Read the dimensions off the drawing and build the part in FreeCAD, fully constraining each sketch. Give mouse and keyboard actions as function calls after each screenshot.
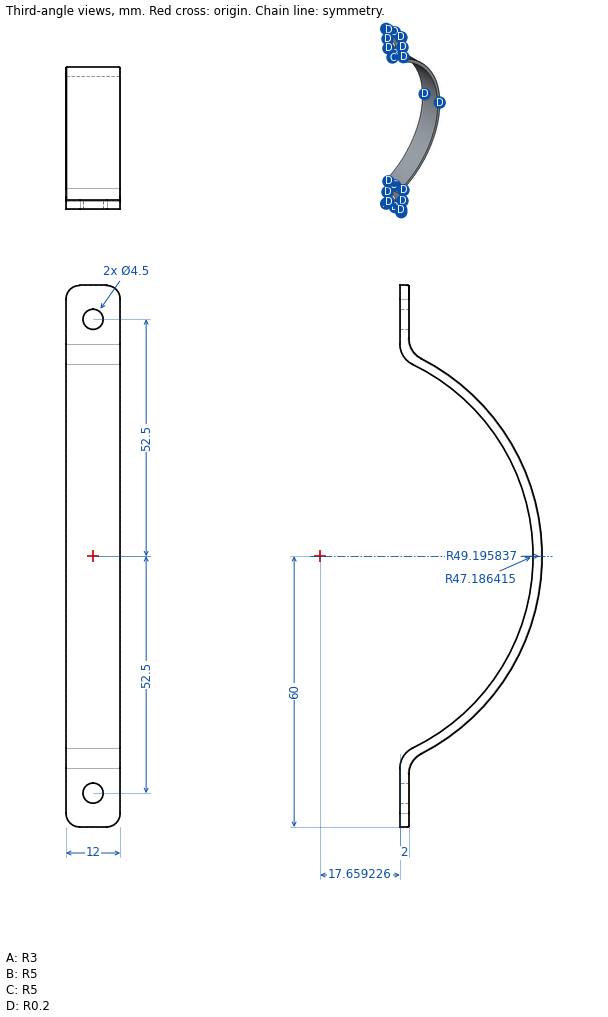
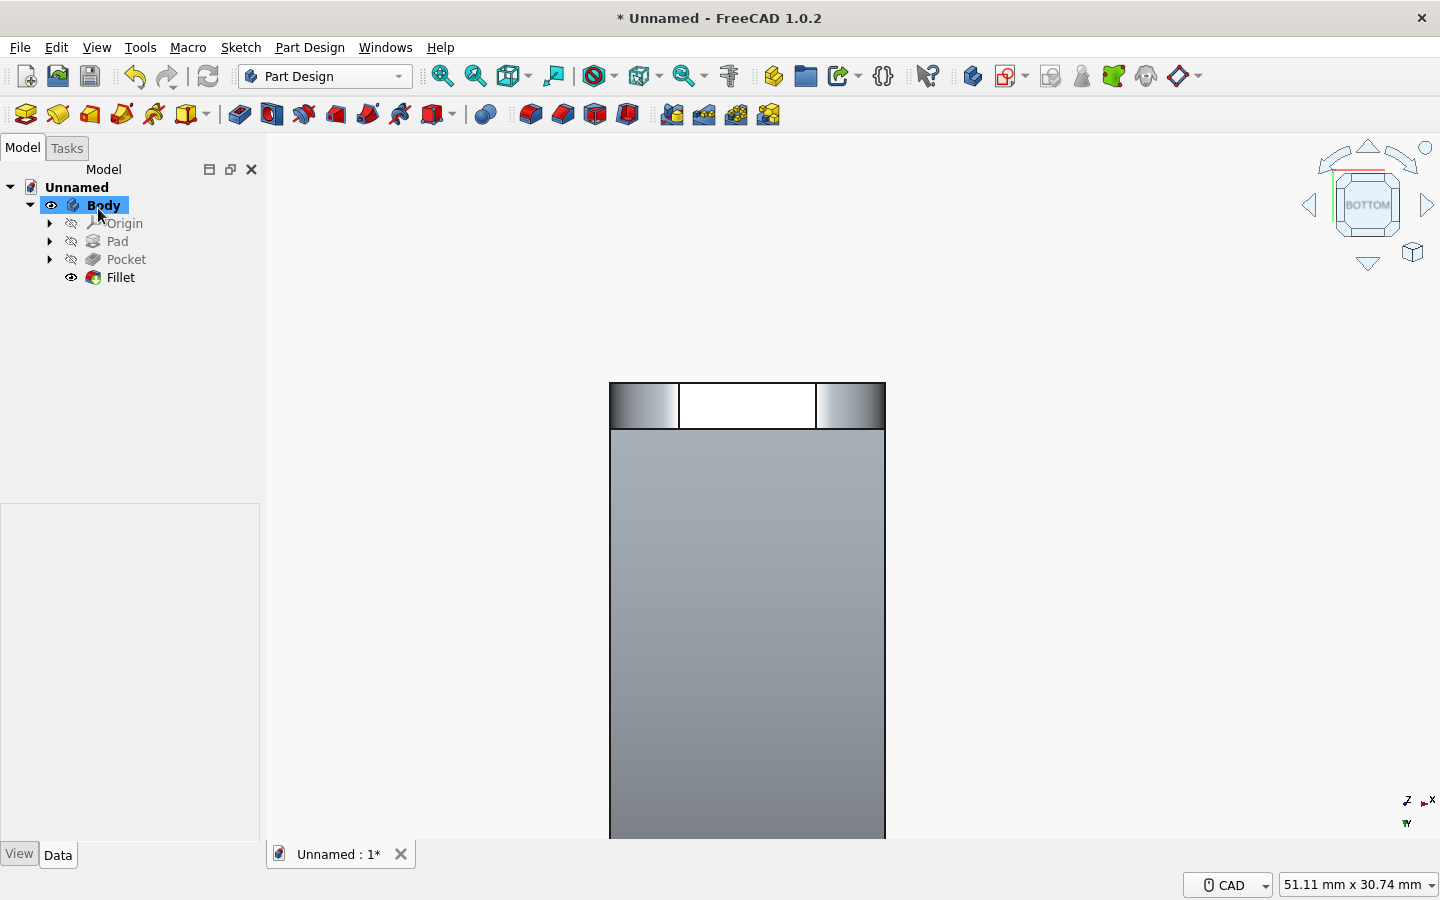
click(444, 76)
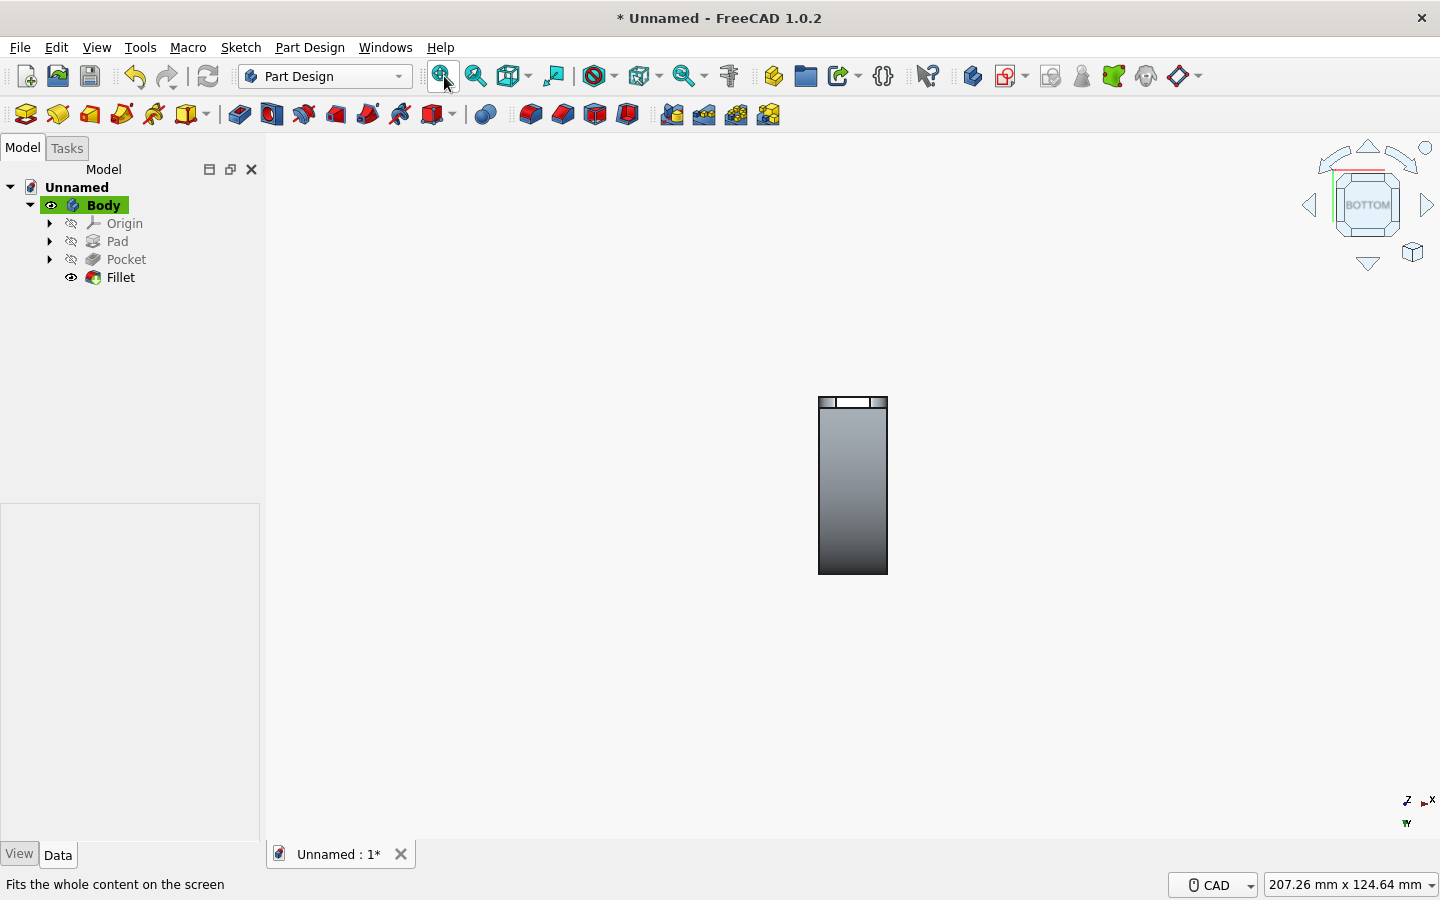
key(0)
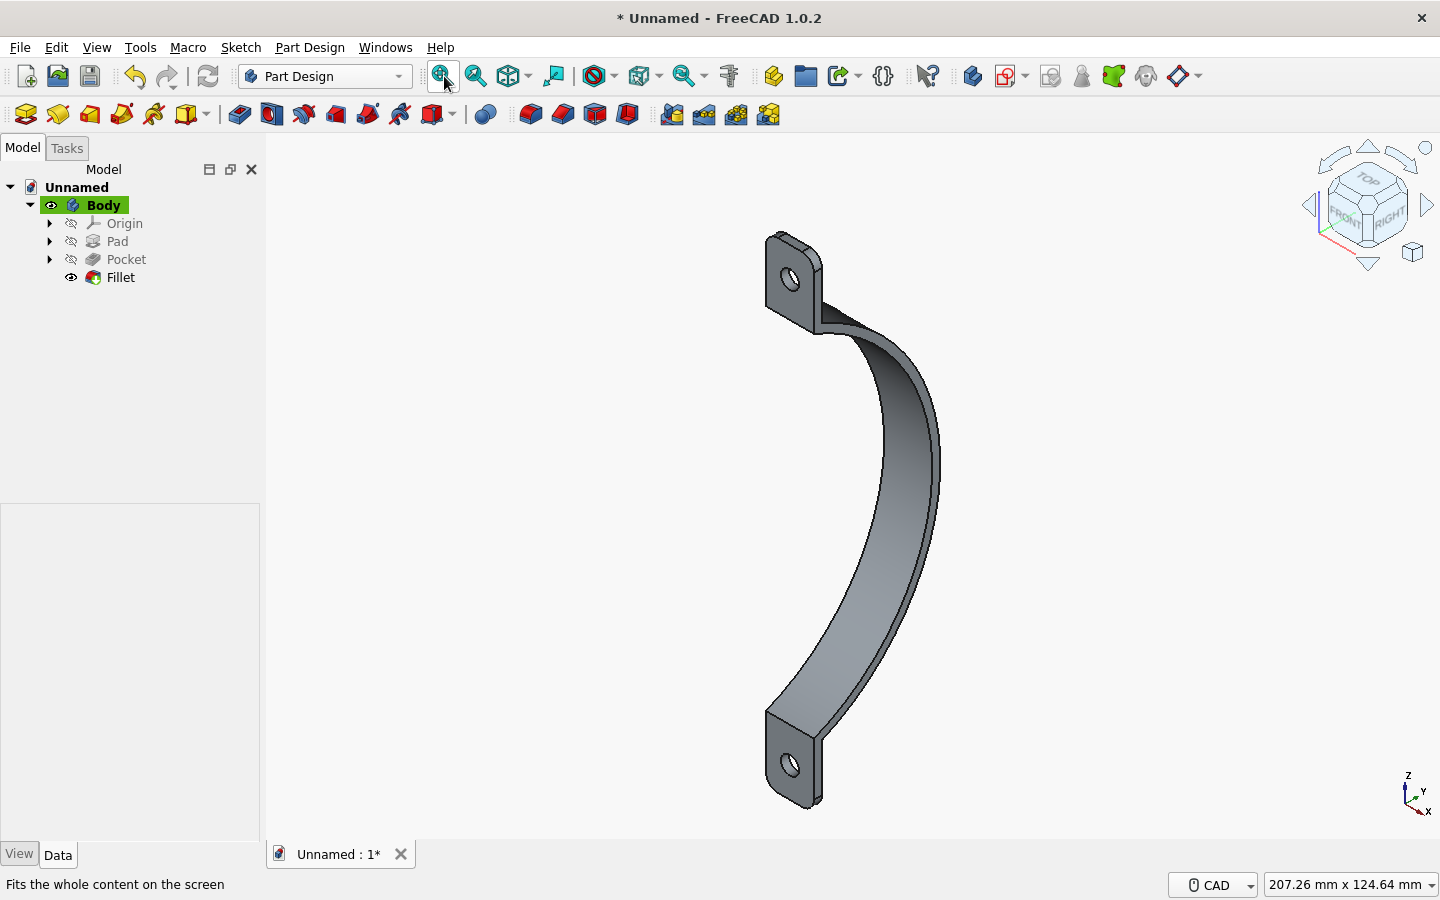
key(2)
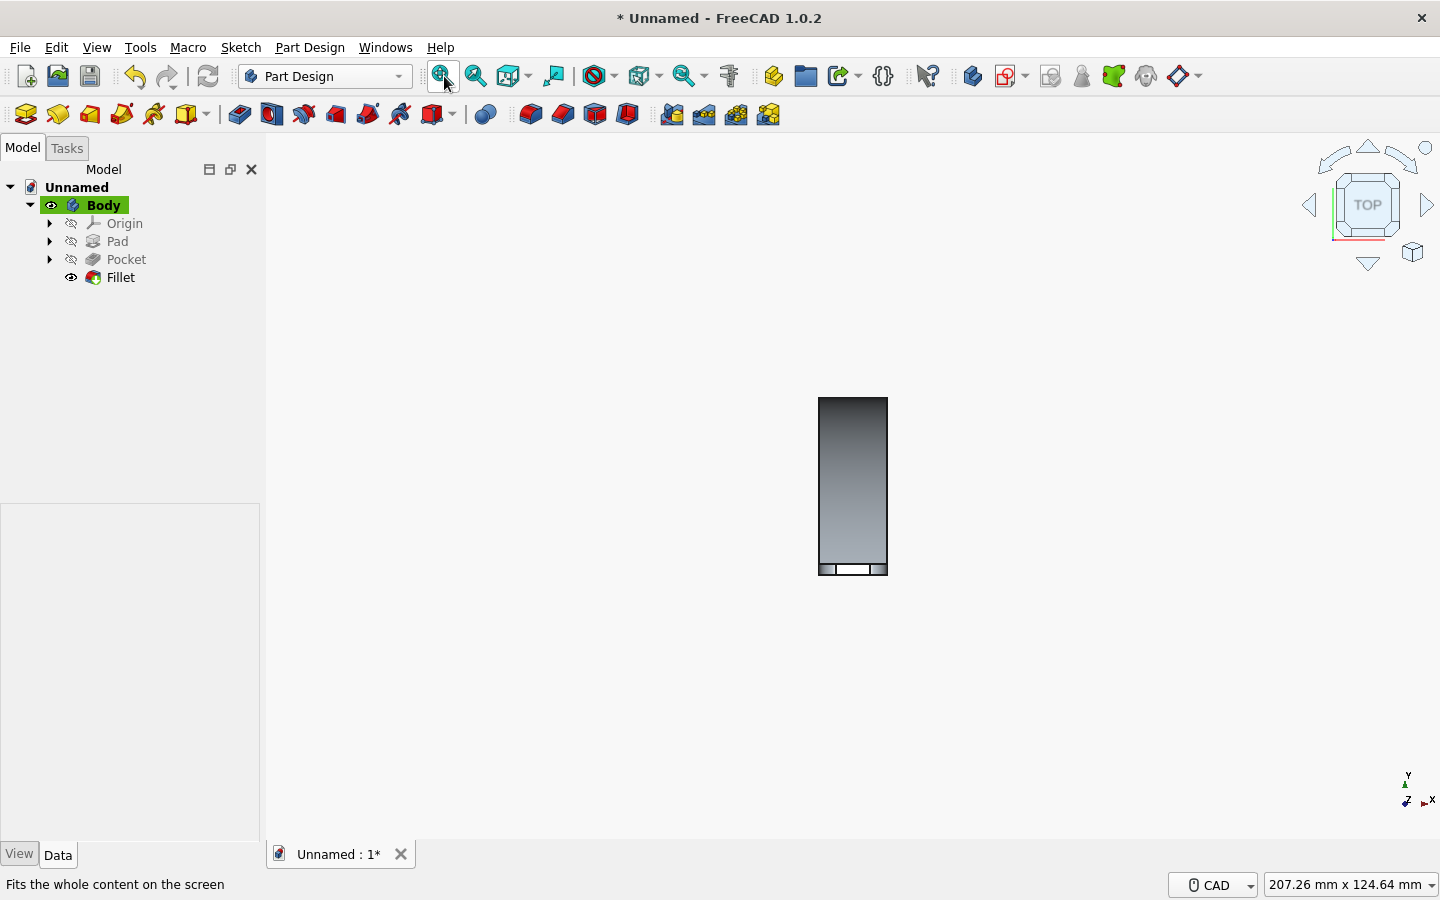
key(v)
key(f)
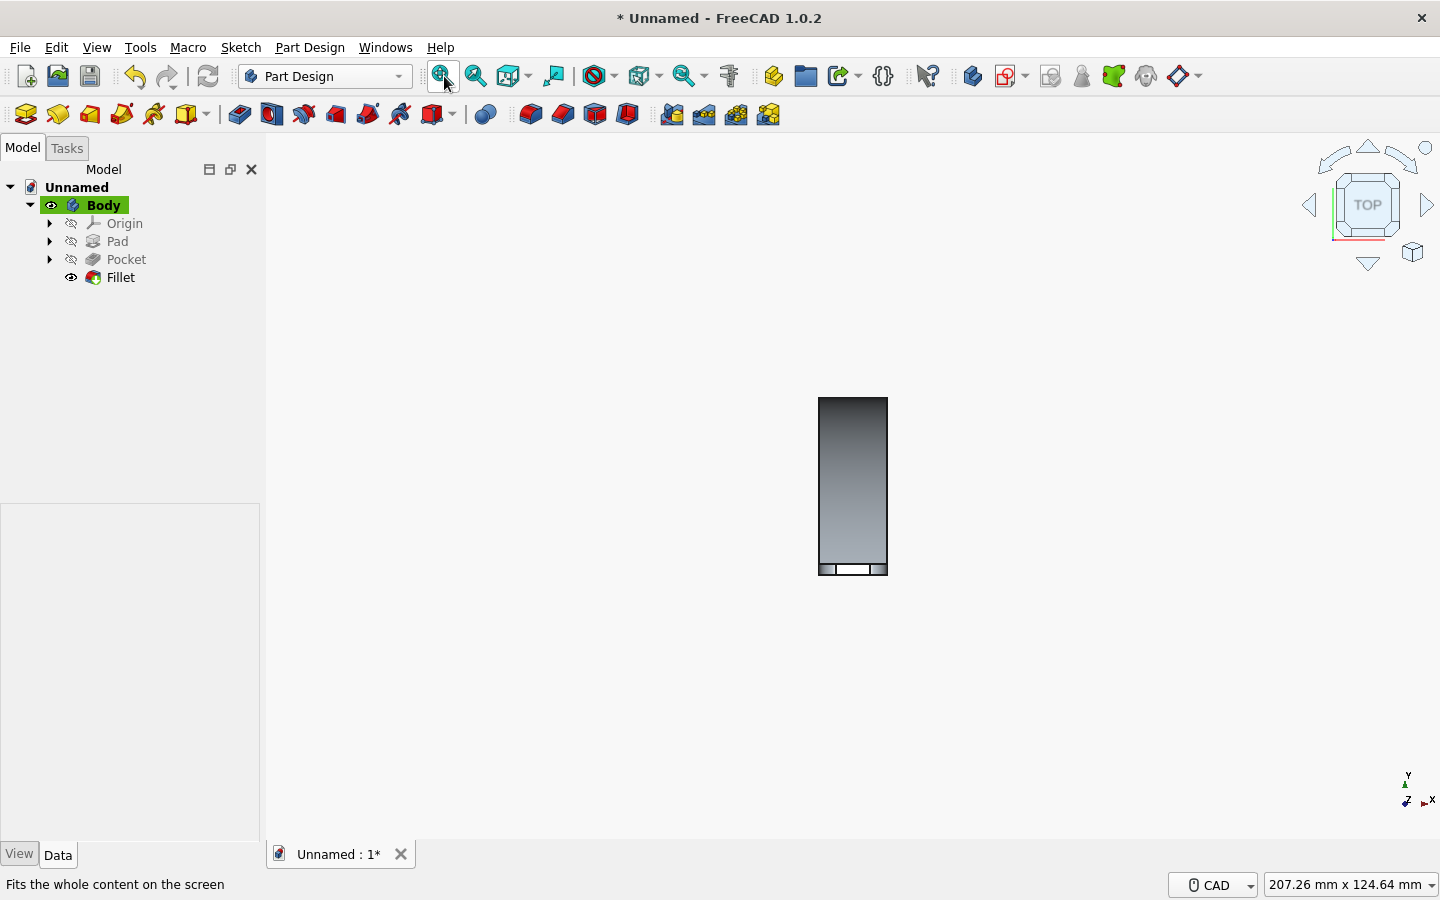
key(1)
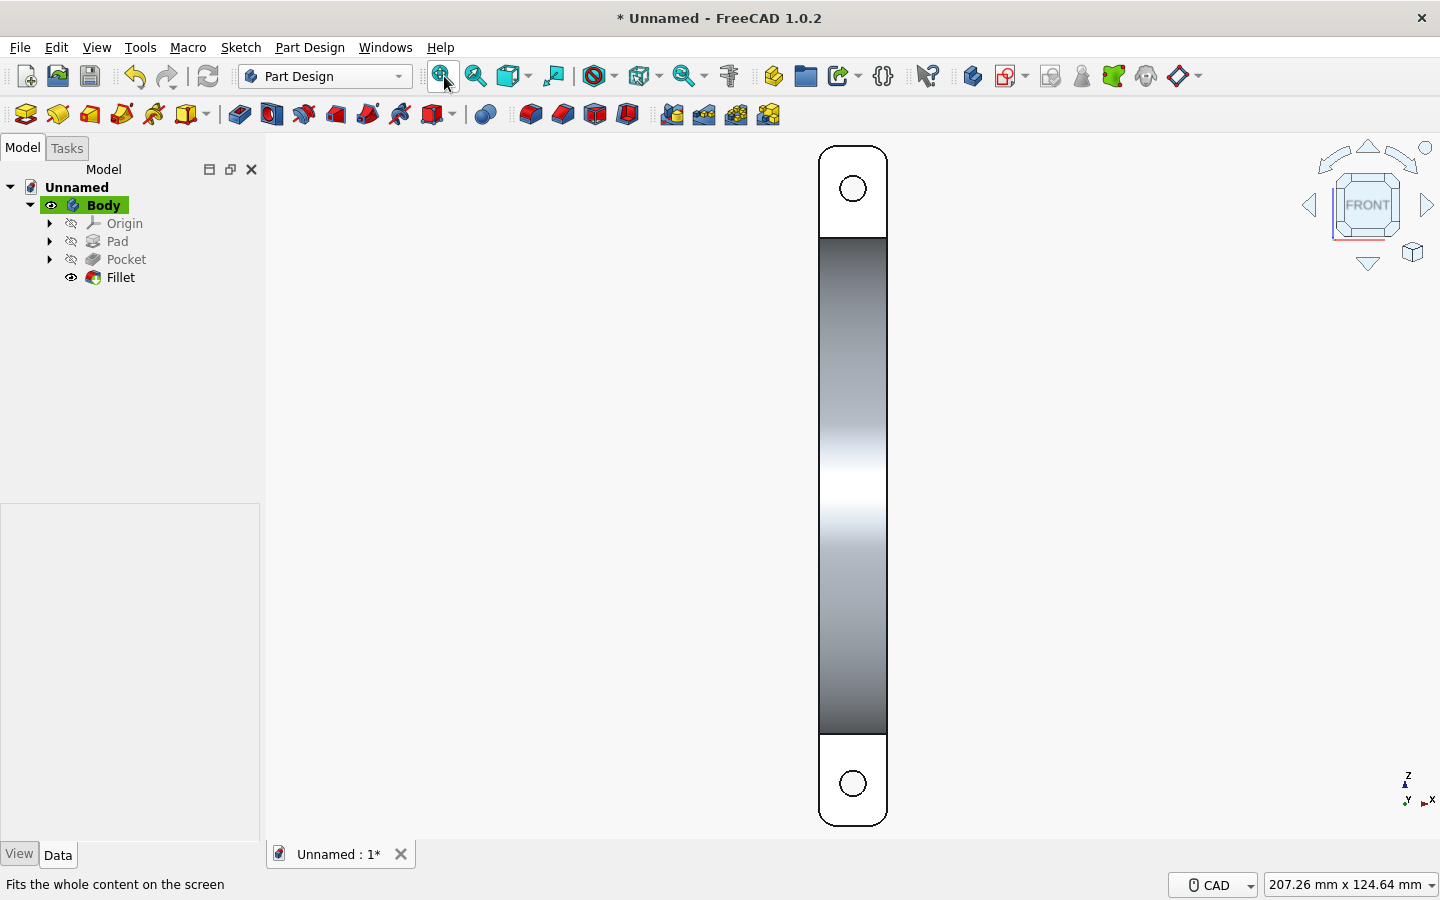
key(3)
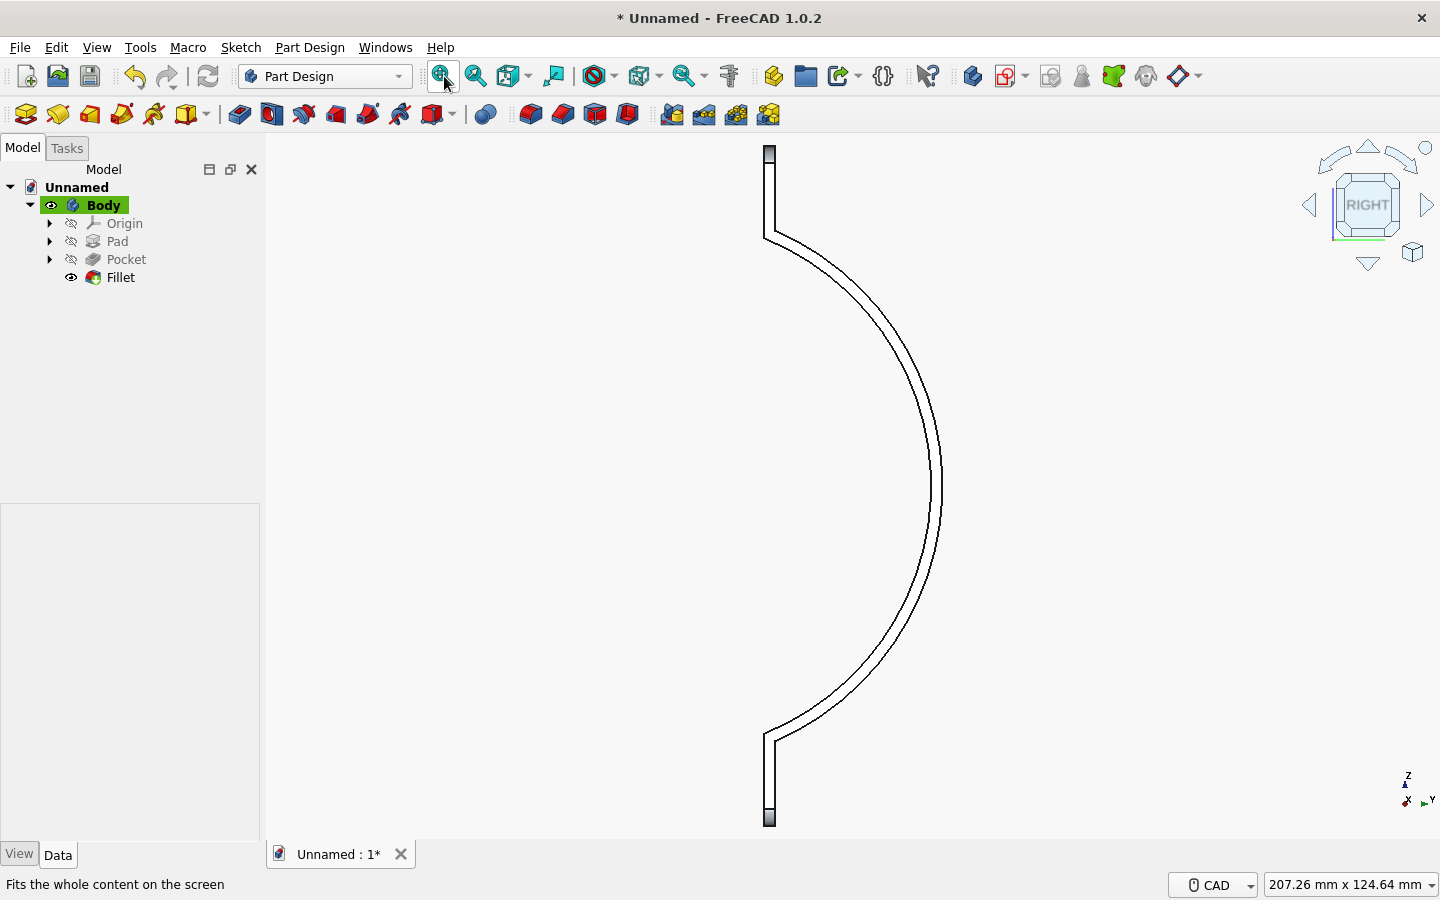
key(5)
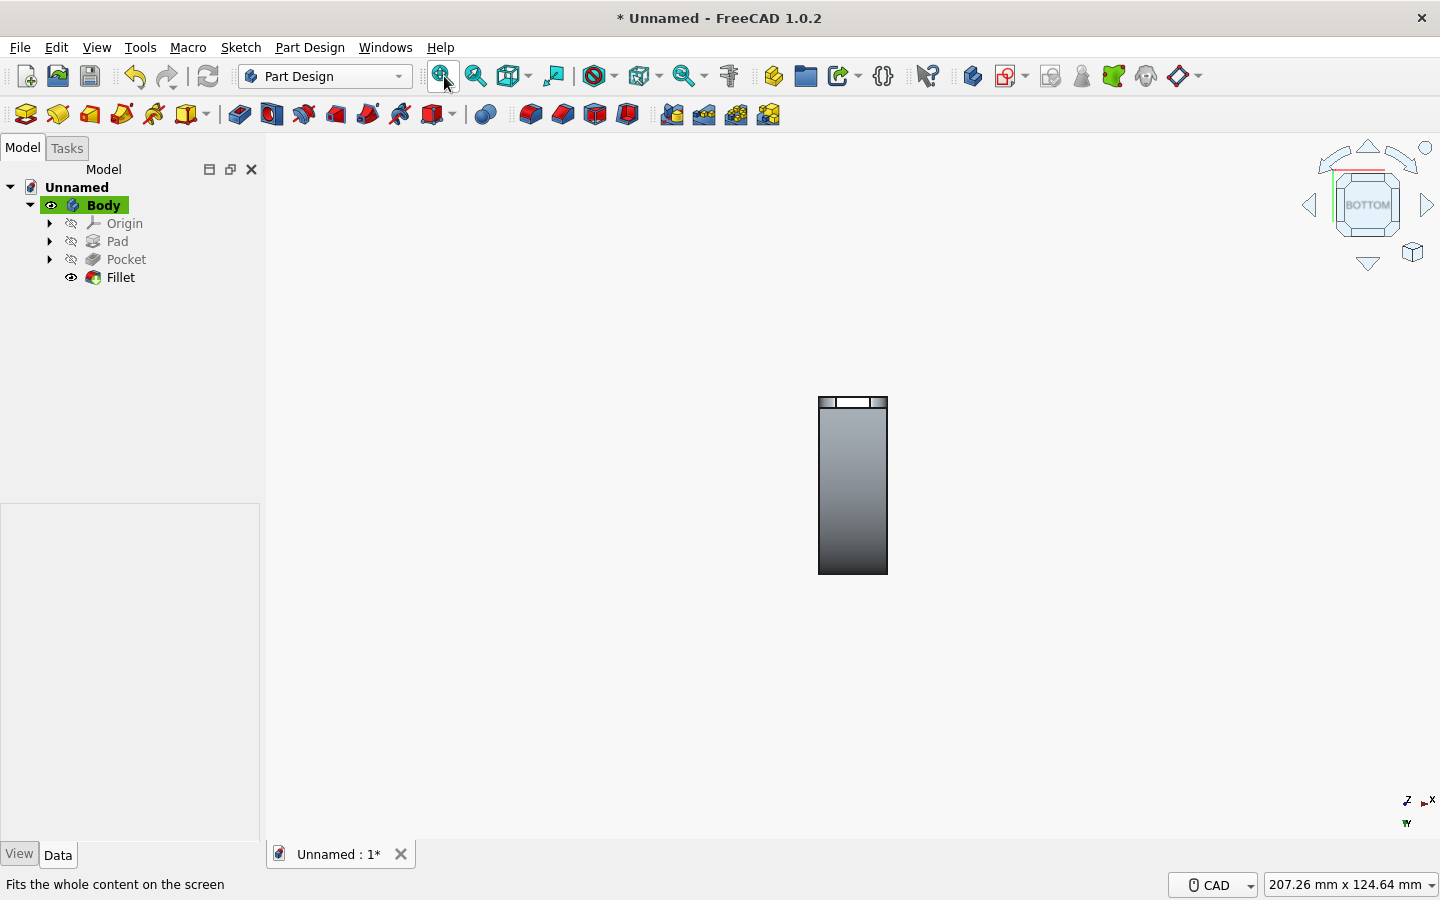
click(444, 76)